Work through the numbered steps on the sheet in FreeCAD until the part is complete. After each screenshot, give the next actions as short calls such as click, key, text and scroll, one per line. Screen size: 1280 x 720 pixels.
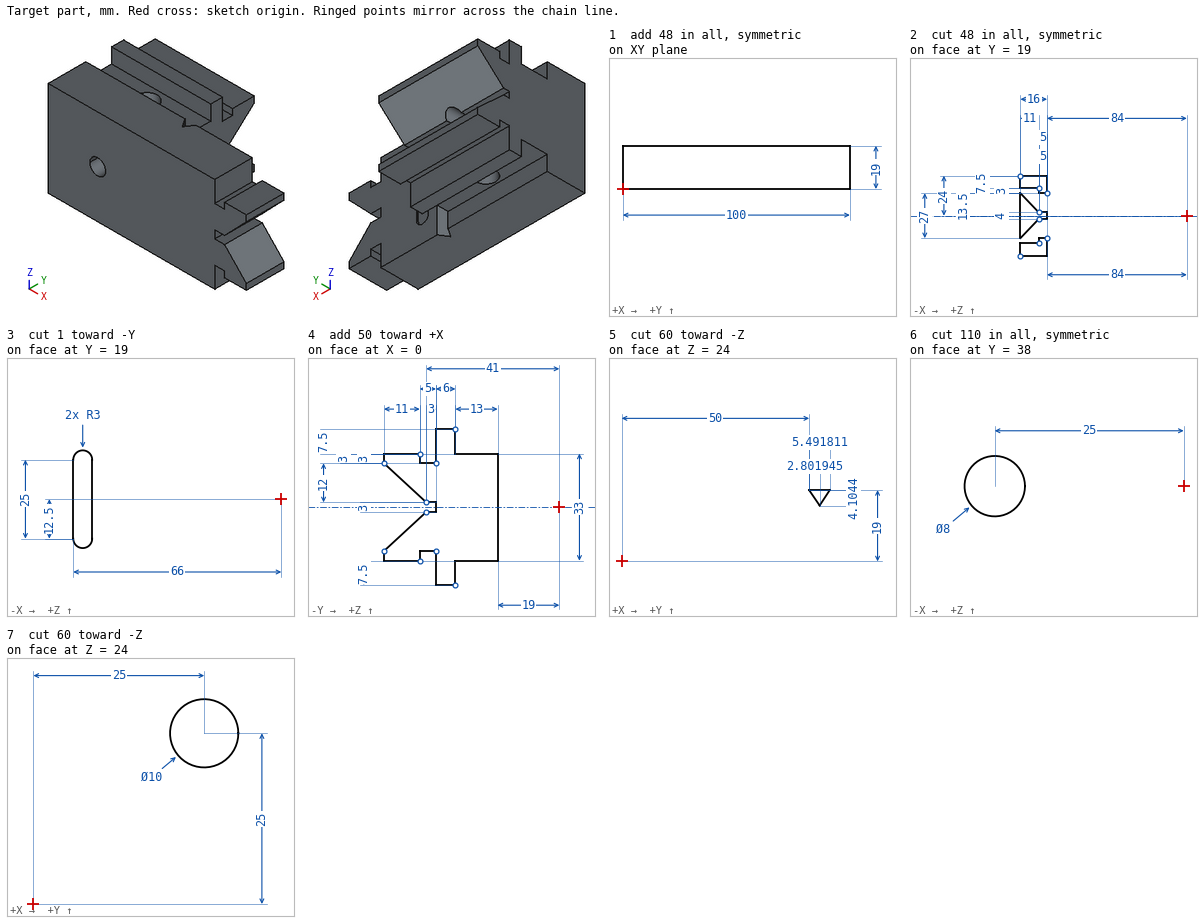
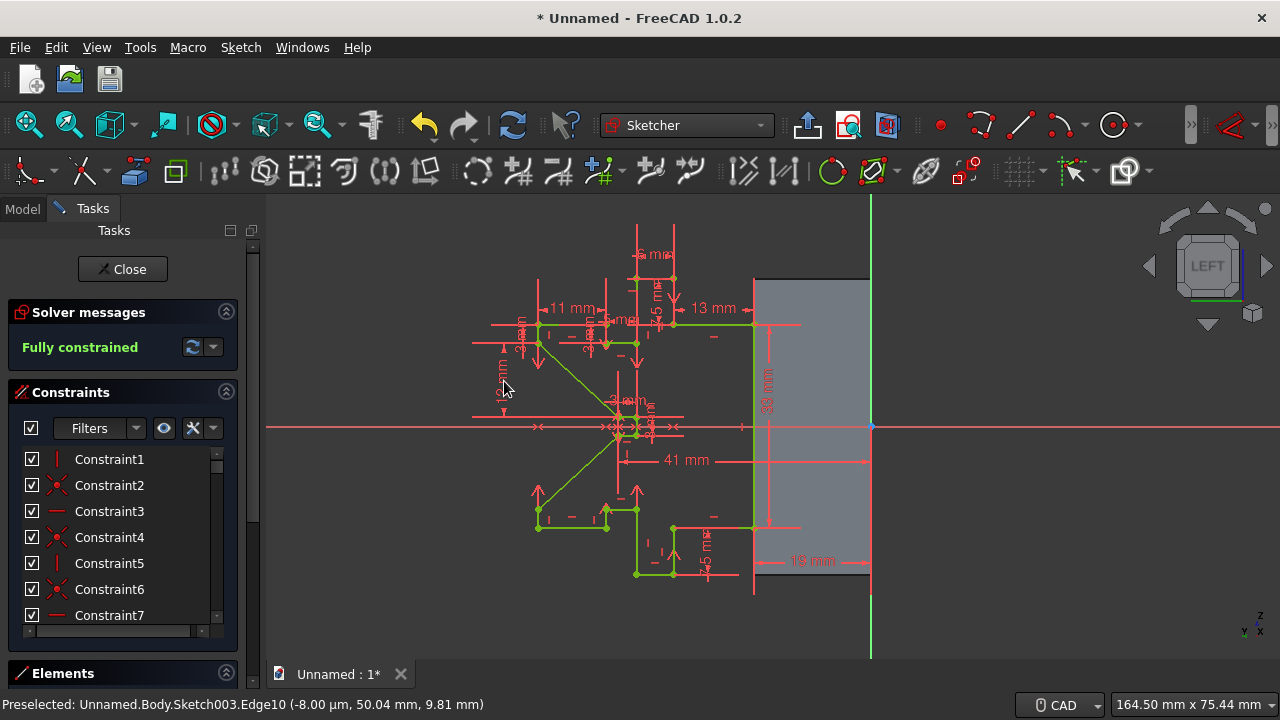
click(123, 269)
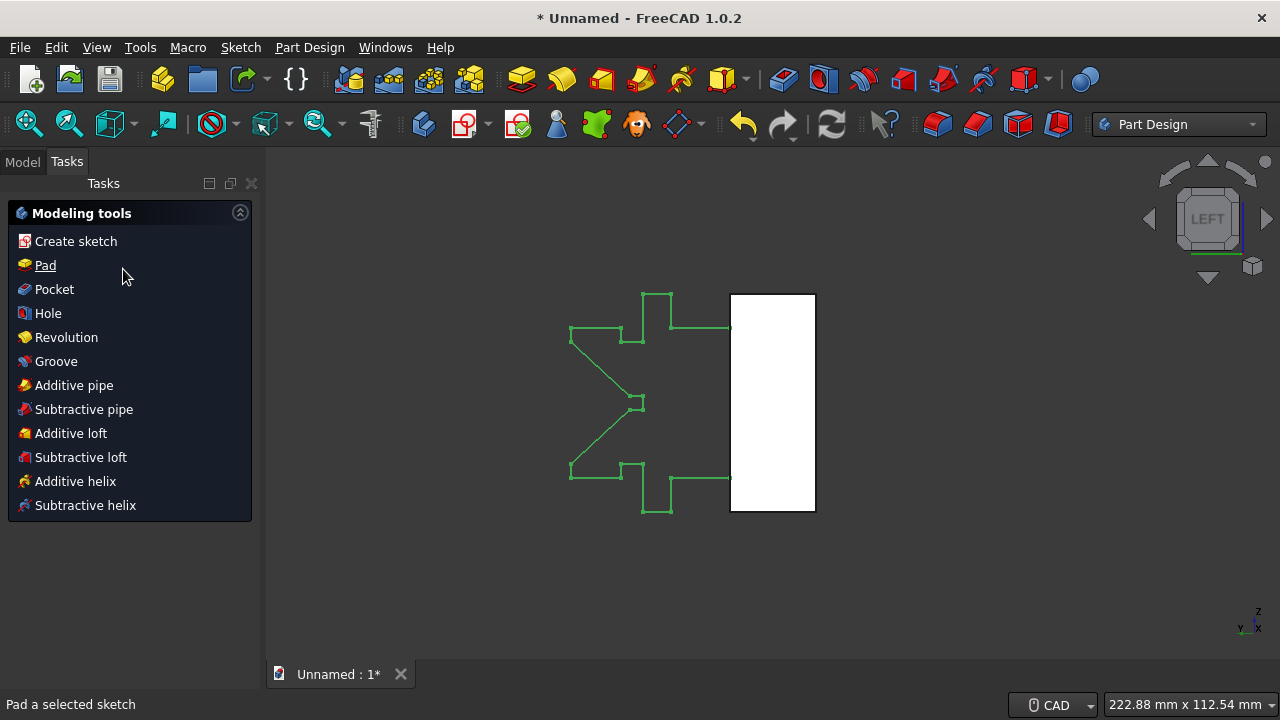
click(522, 80)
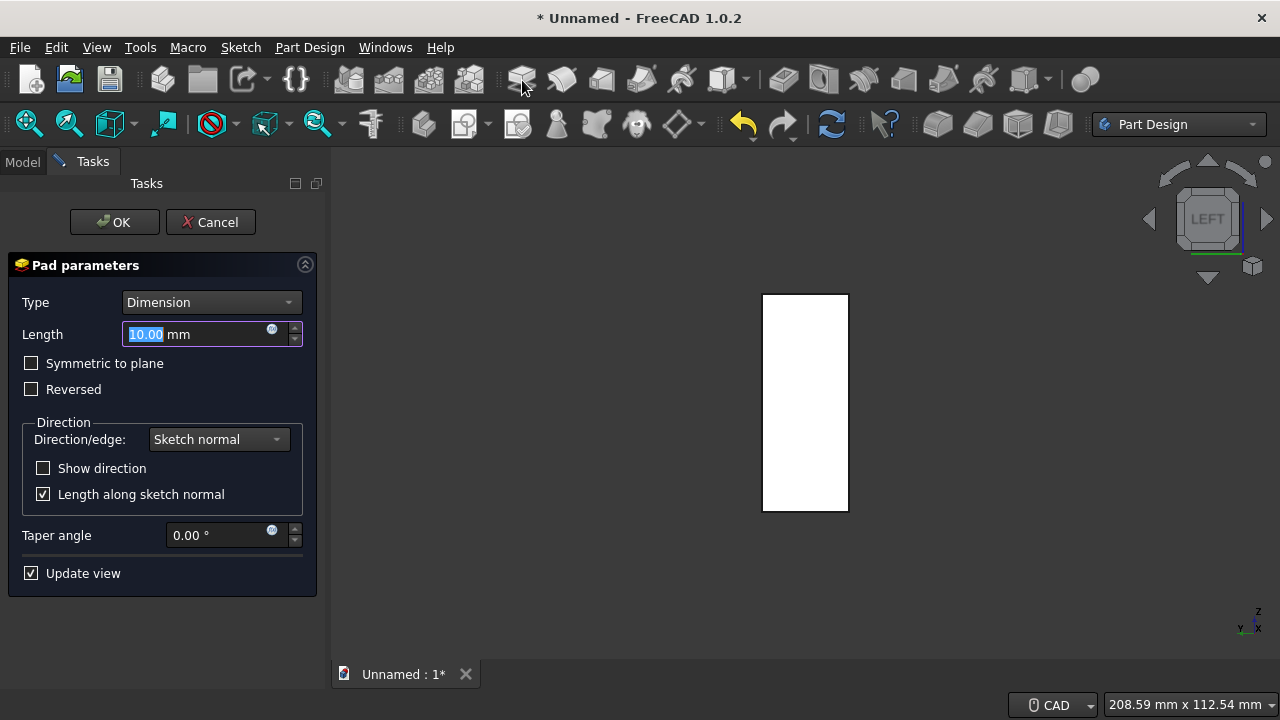
text(50)
key(Tab)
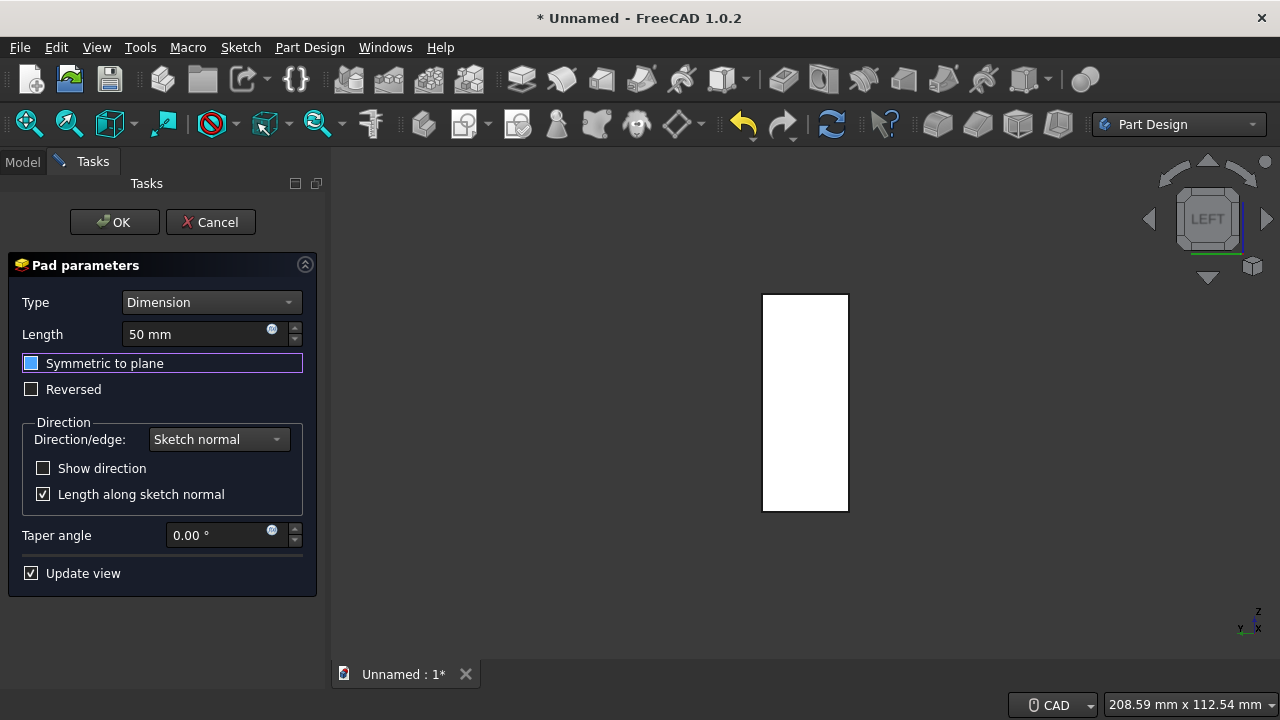
click(30, 389)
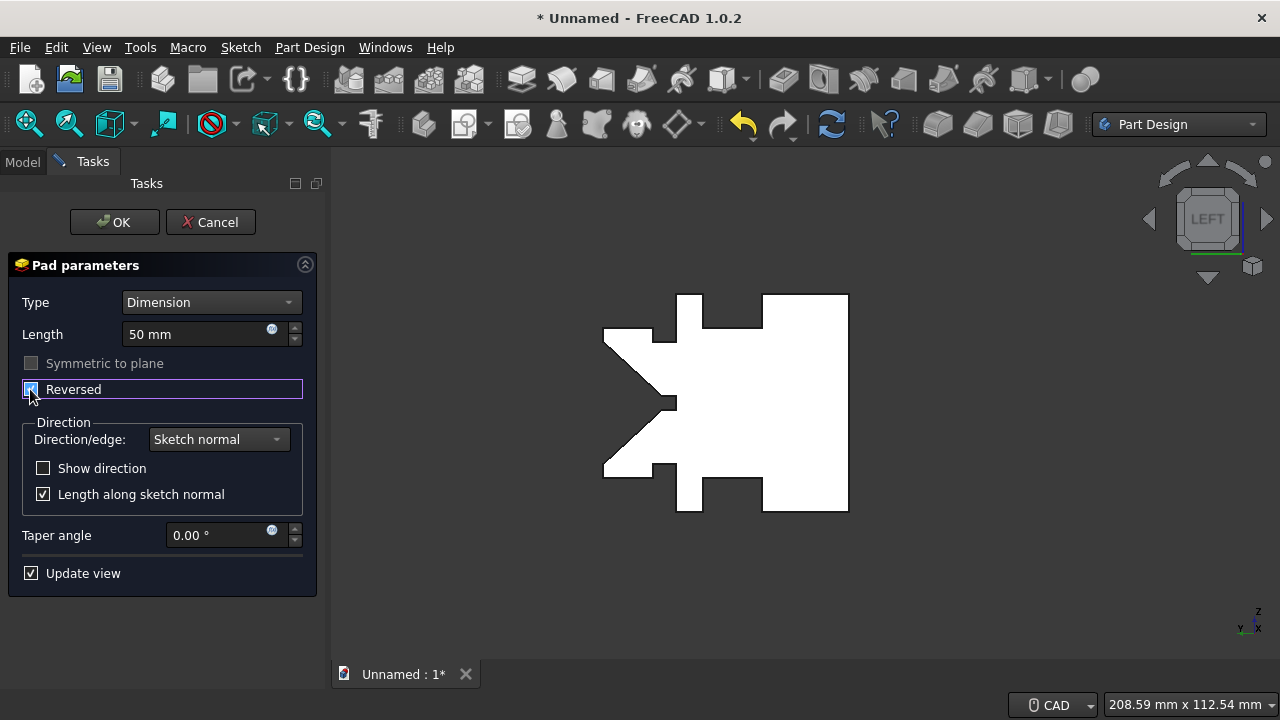
click(115, 222)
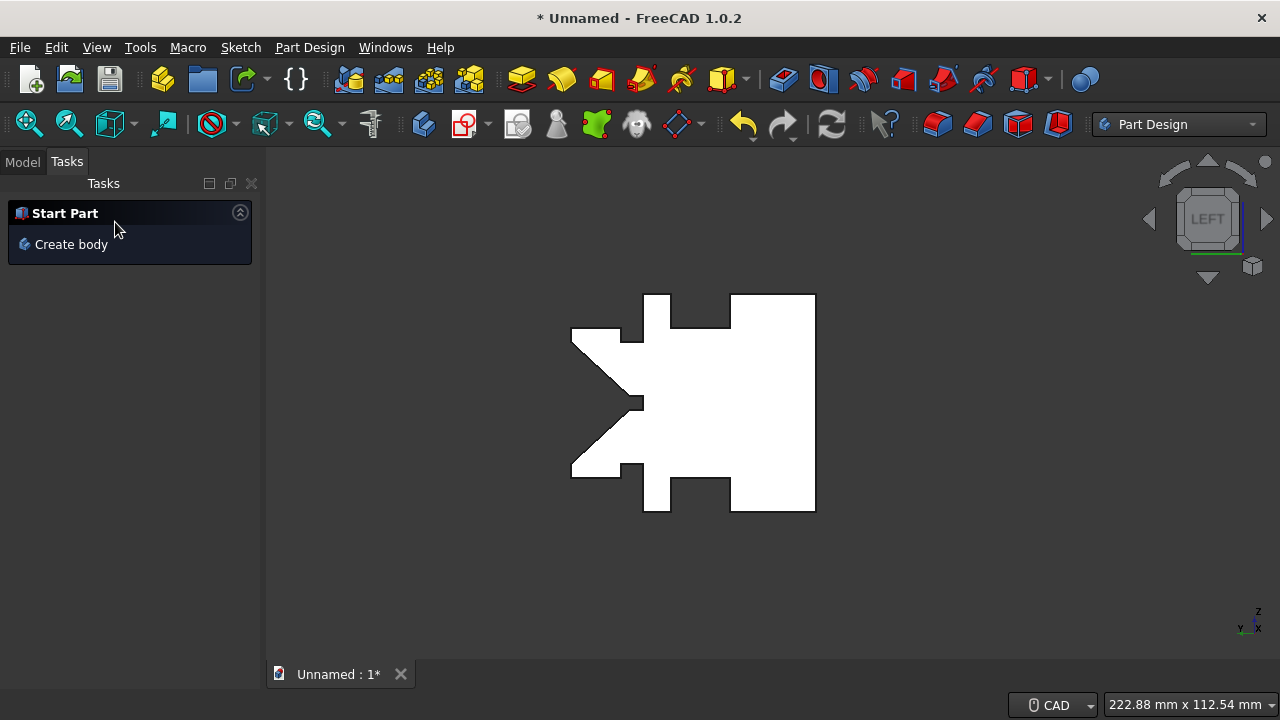
click(30, 124)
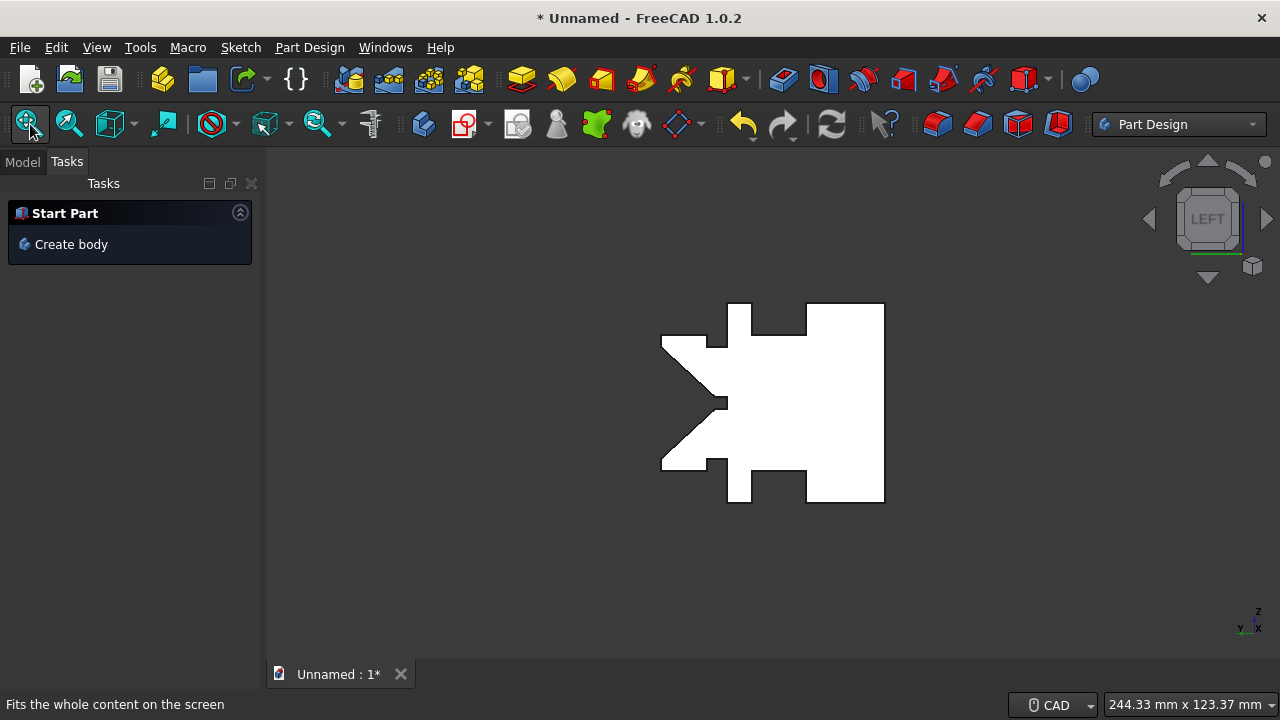
key(0)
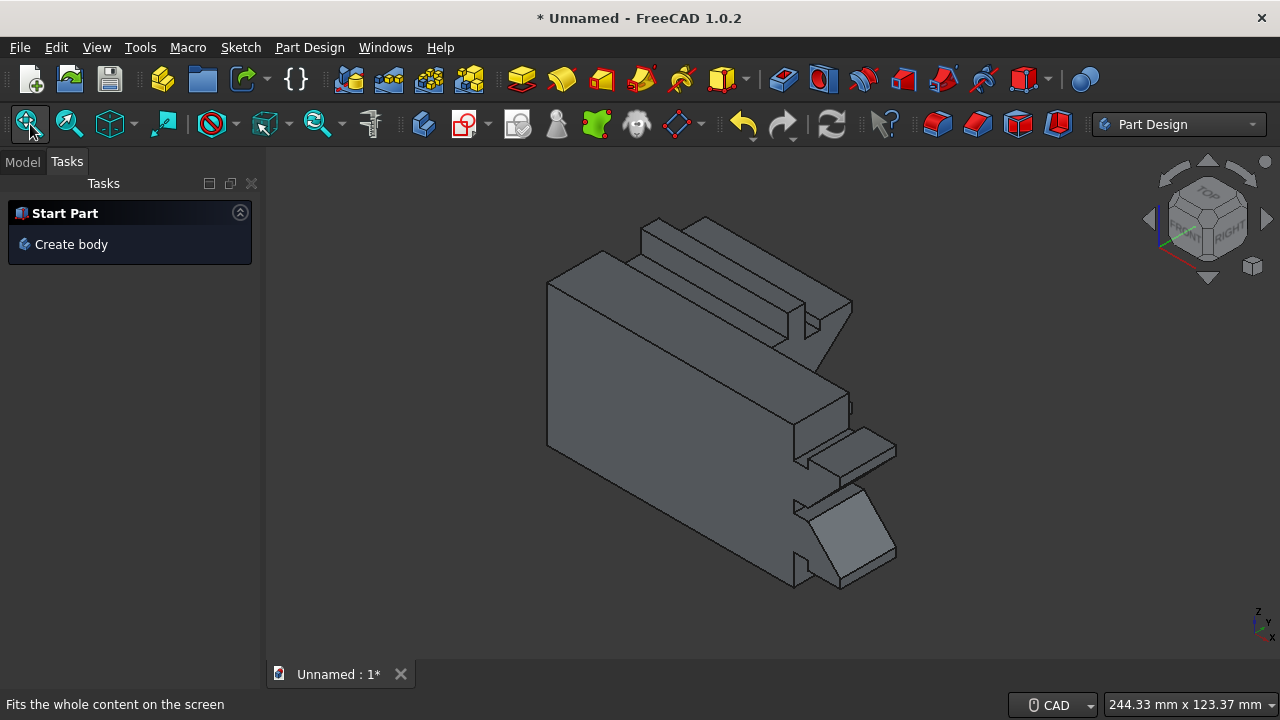
click(769, 377)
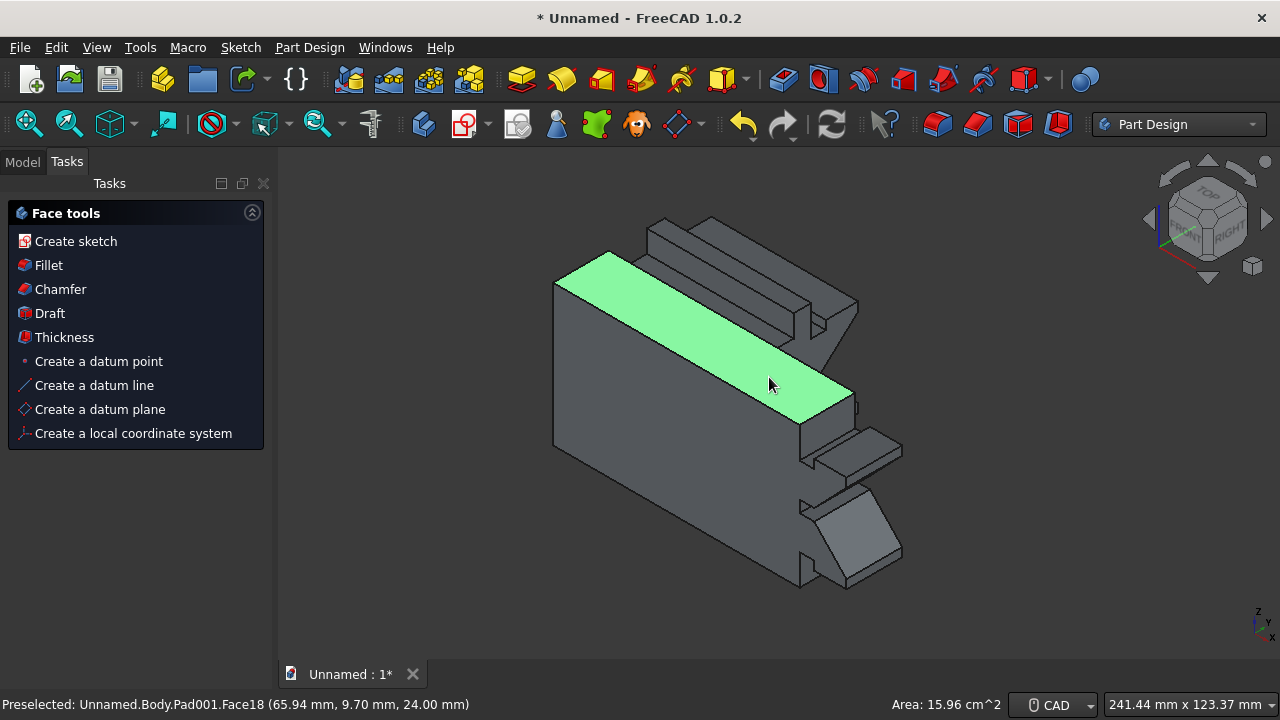
click(464, 124)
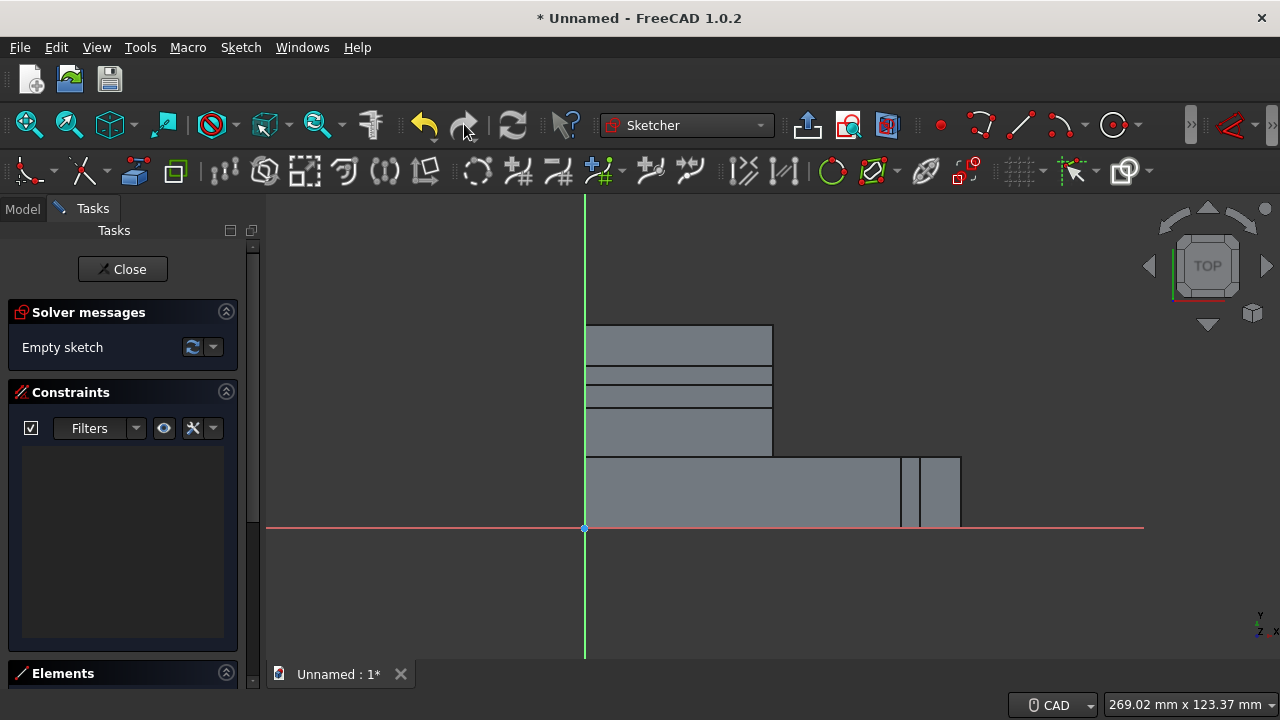
scroll(787, 466, up, 15)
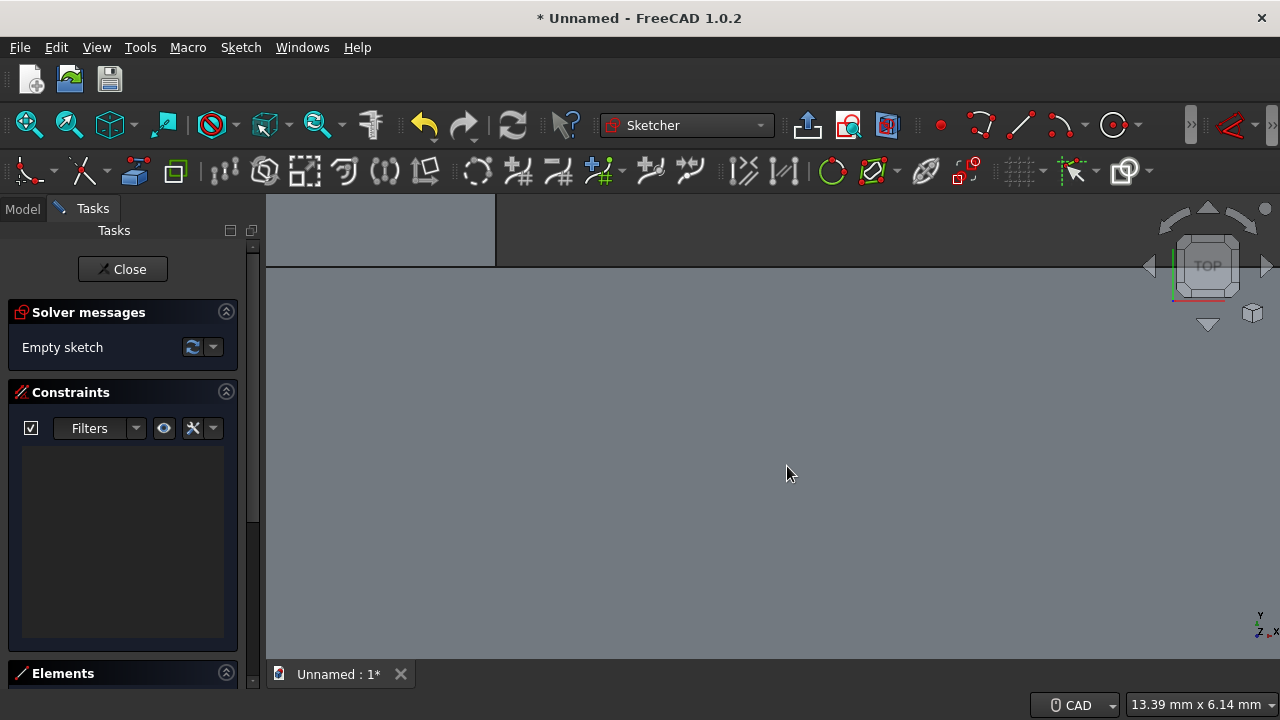
click(982, 126)